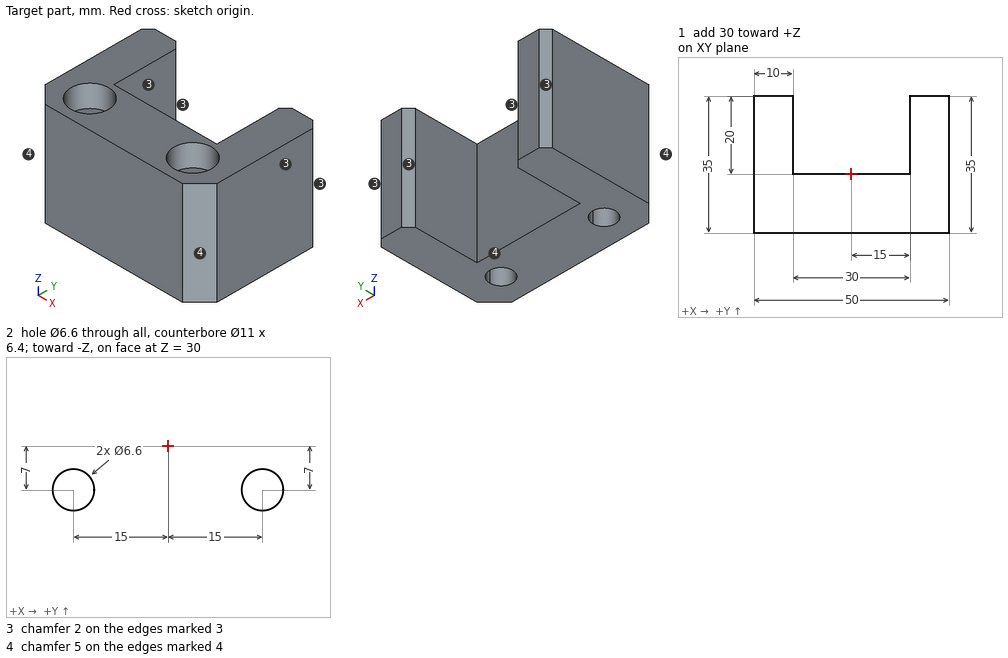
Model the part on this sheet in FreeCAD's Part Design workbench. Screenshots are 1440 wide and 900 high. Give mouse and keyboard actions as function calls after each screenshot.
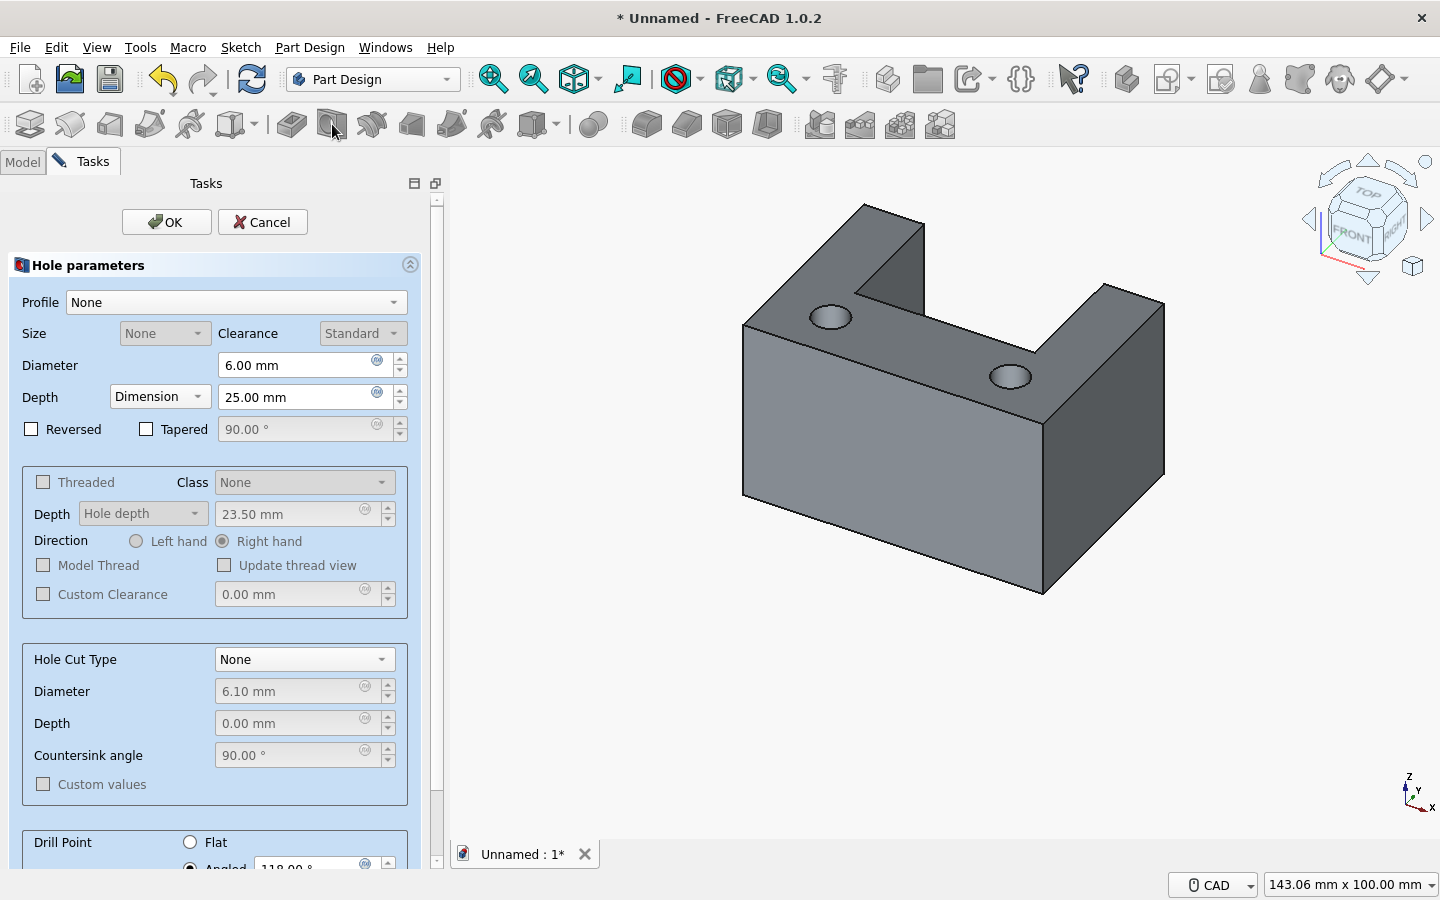
triple_click(305, 365)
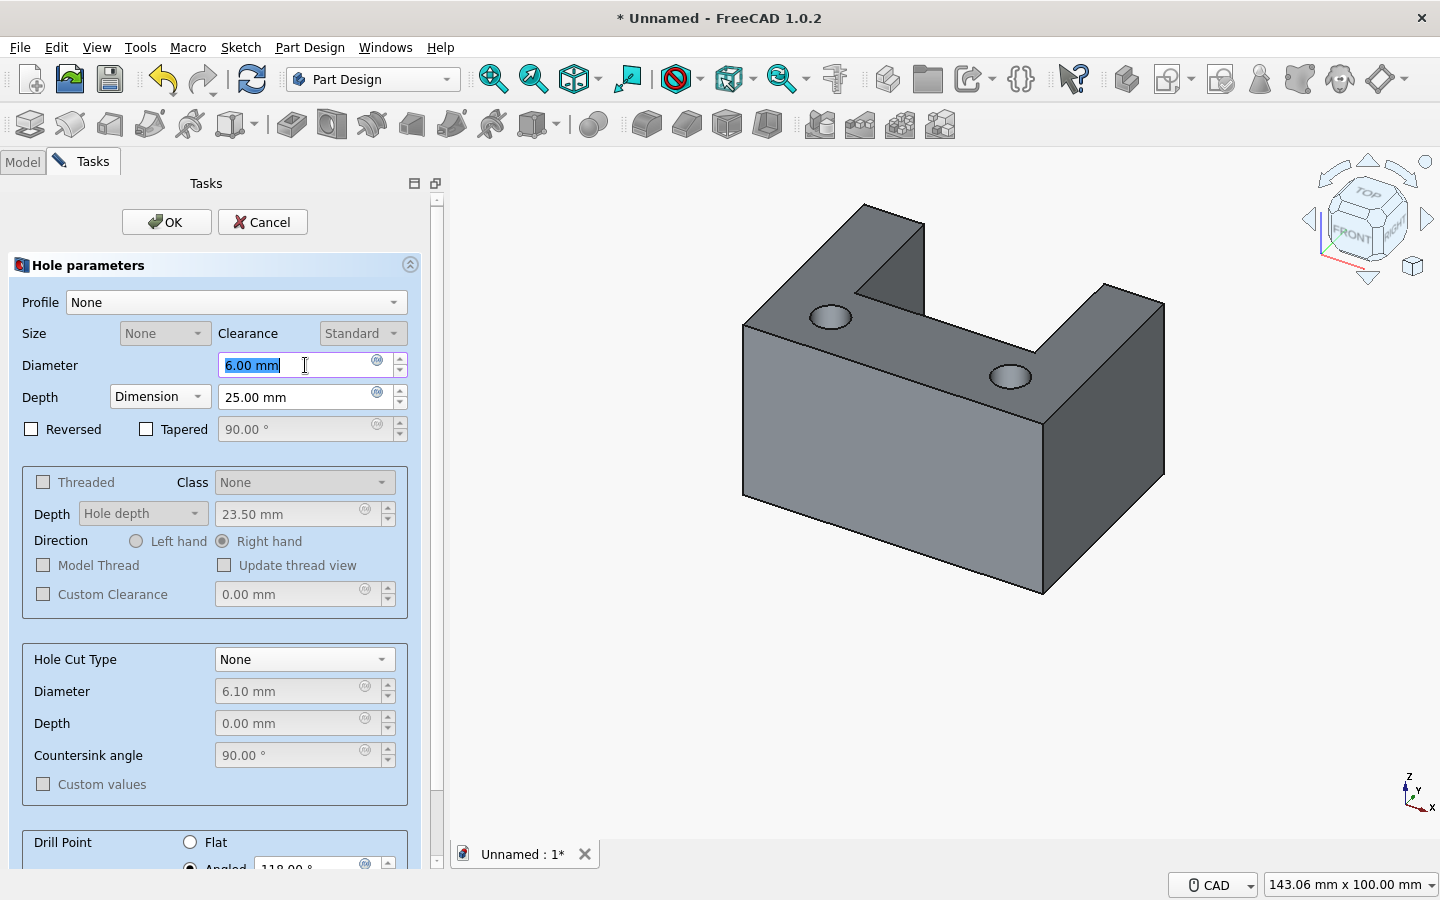
text(6.6)
key(Tab)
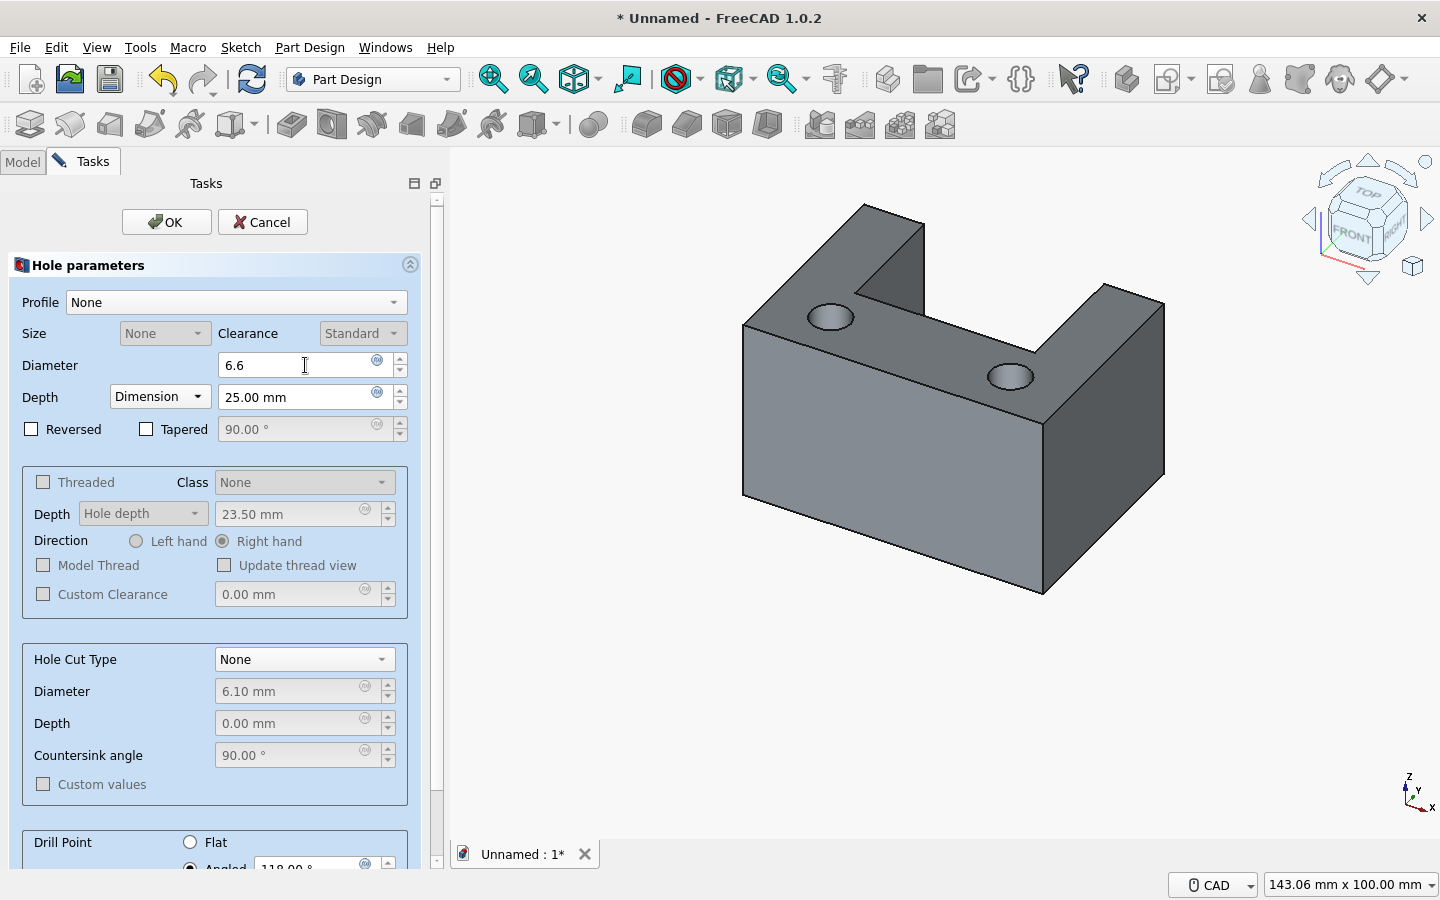
click(161, 396)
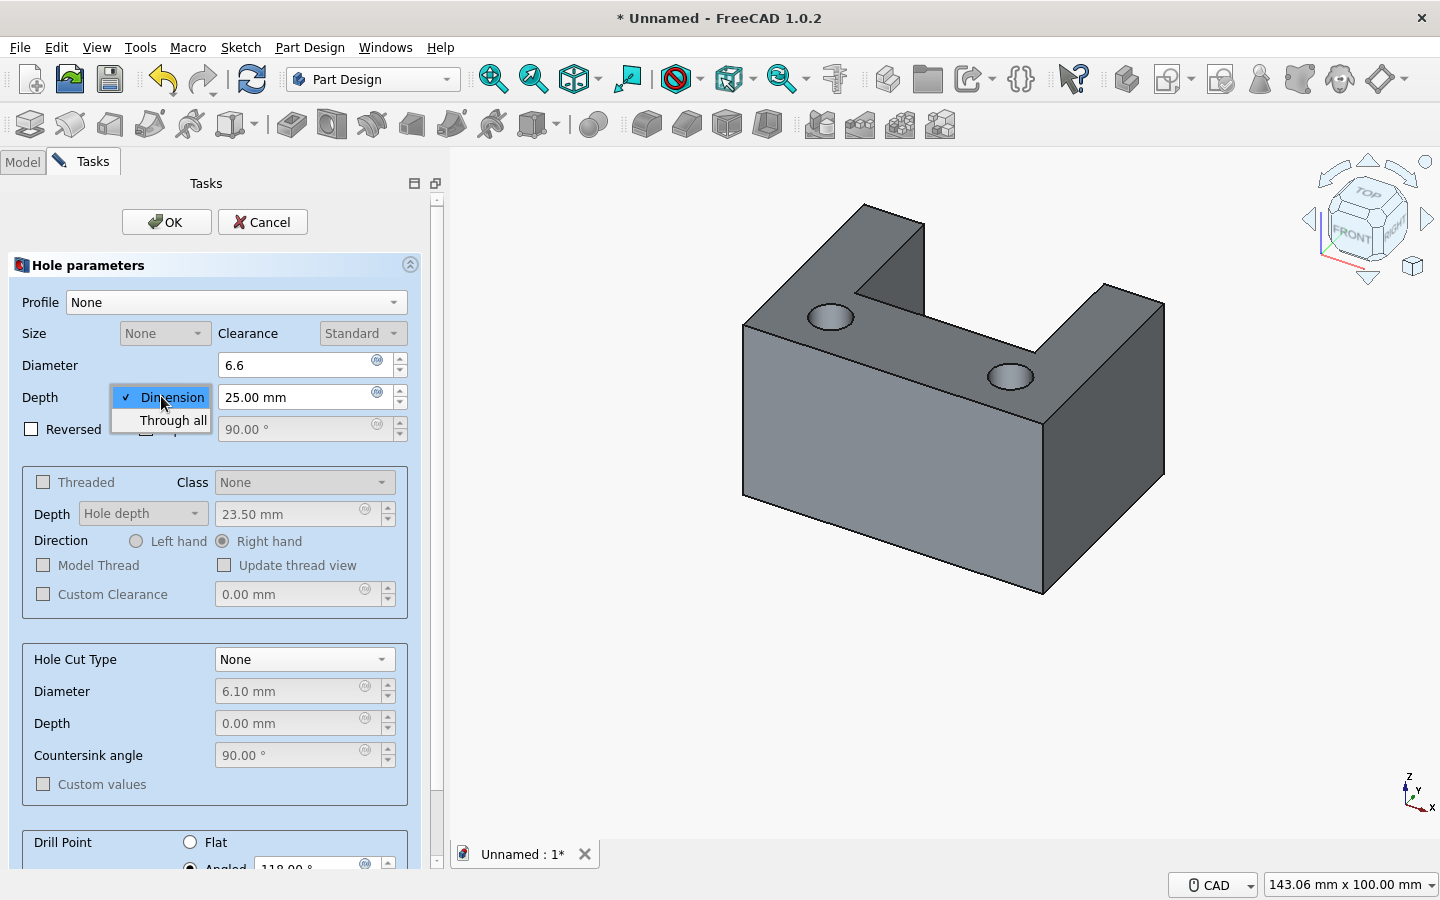
click(160, 420)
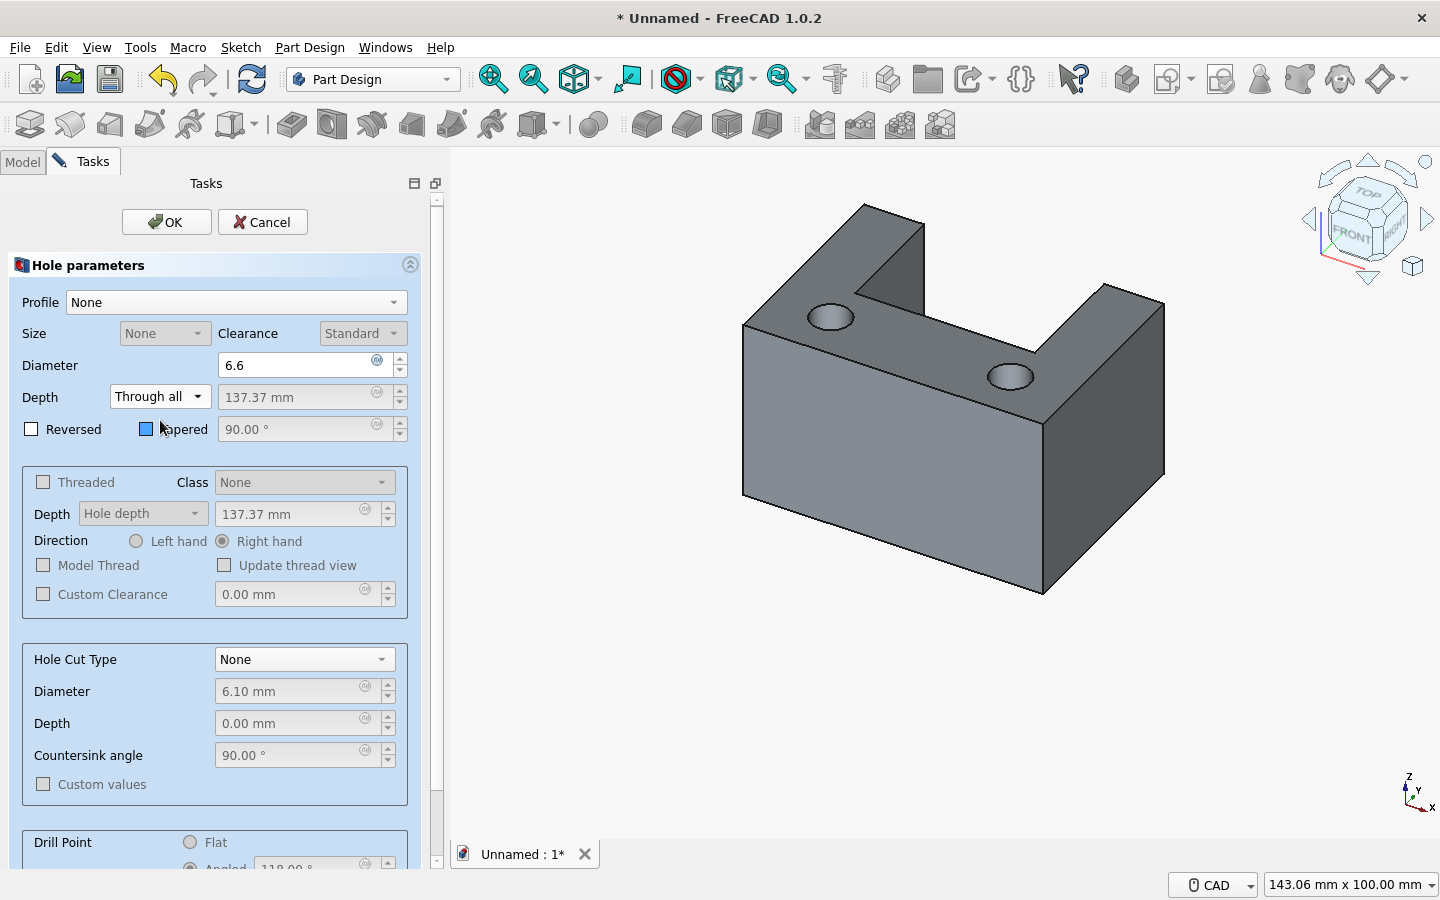
click(306, 660)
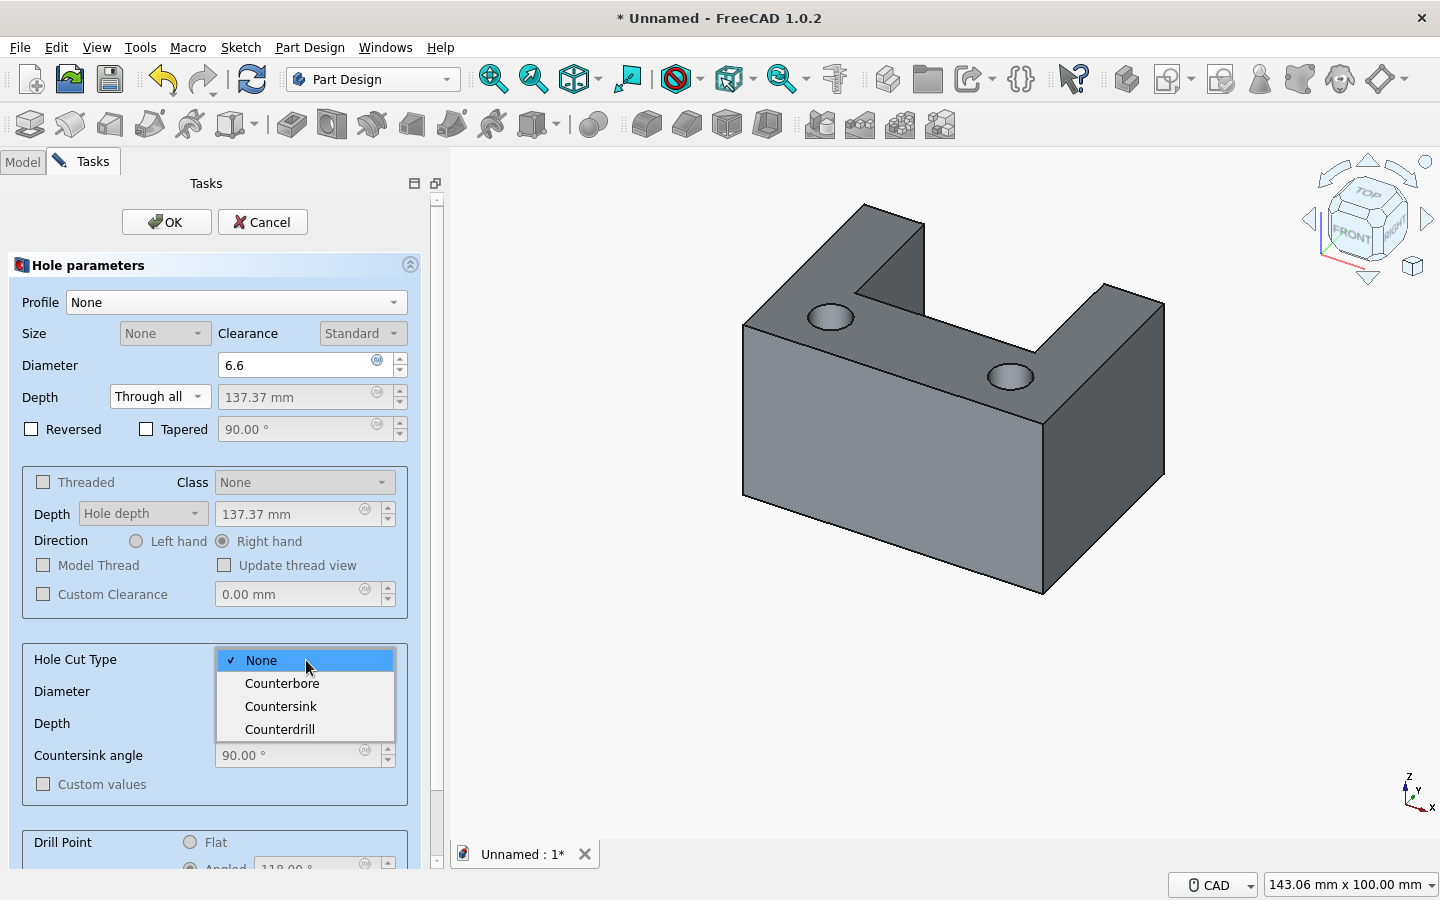
click(304, 684)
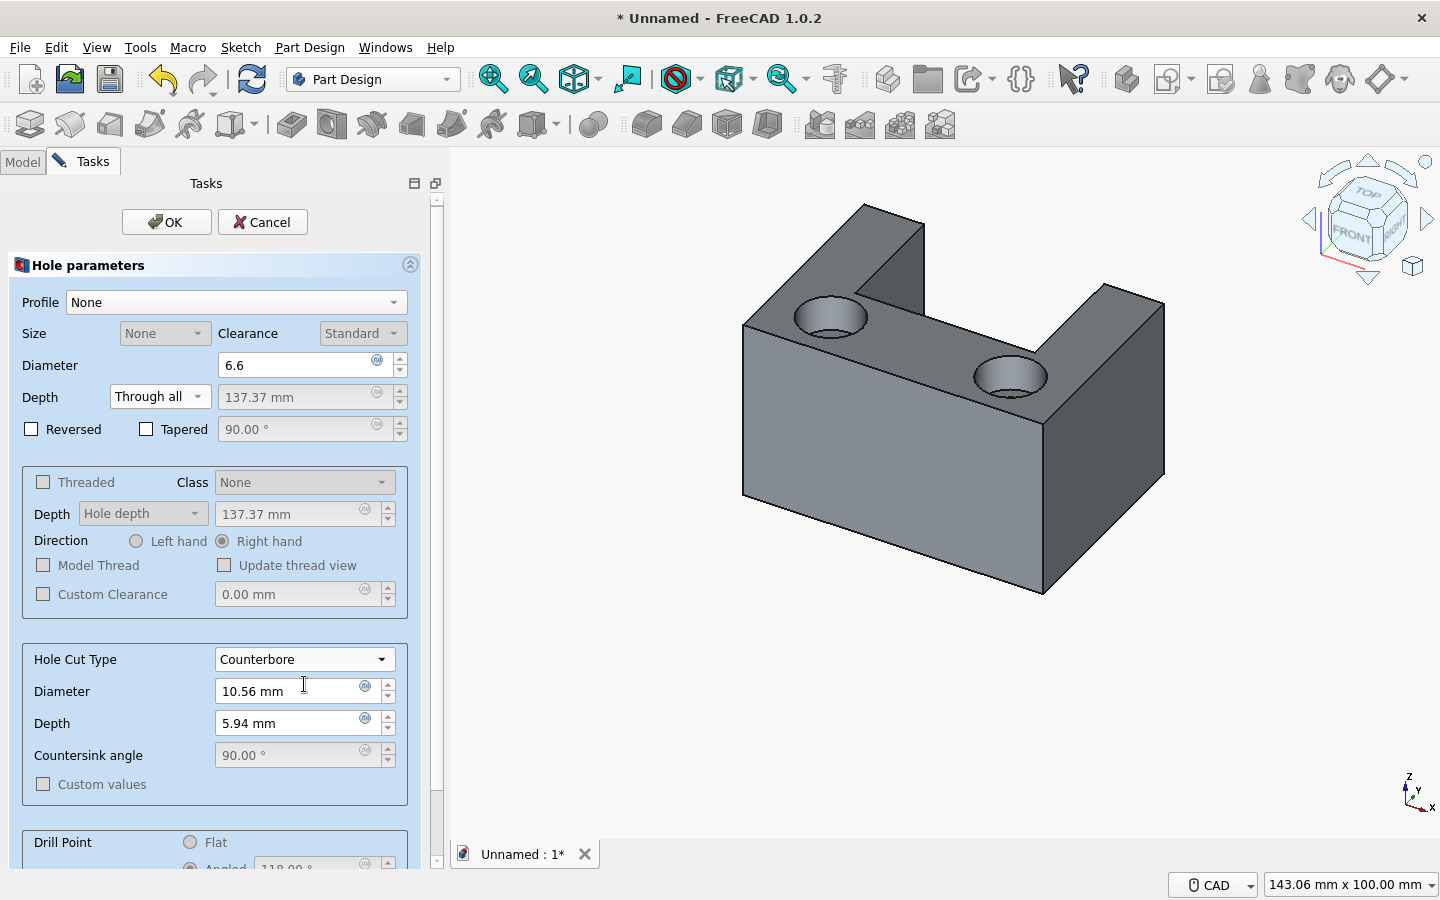
triple_click(298, 691)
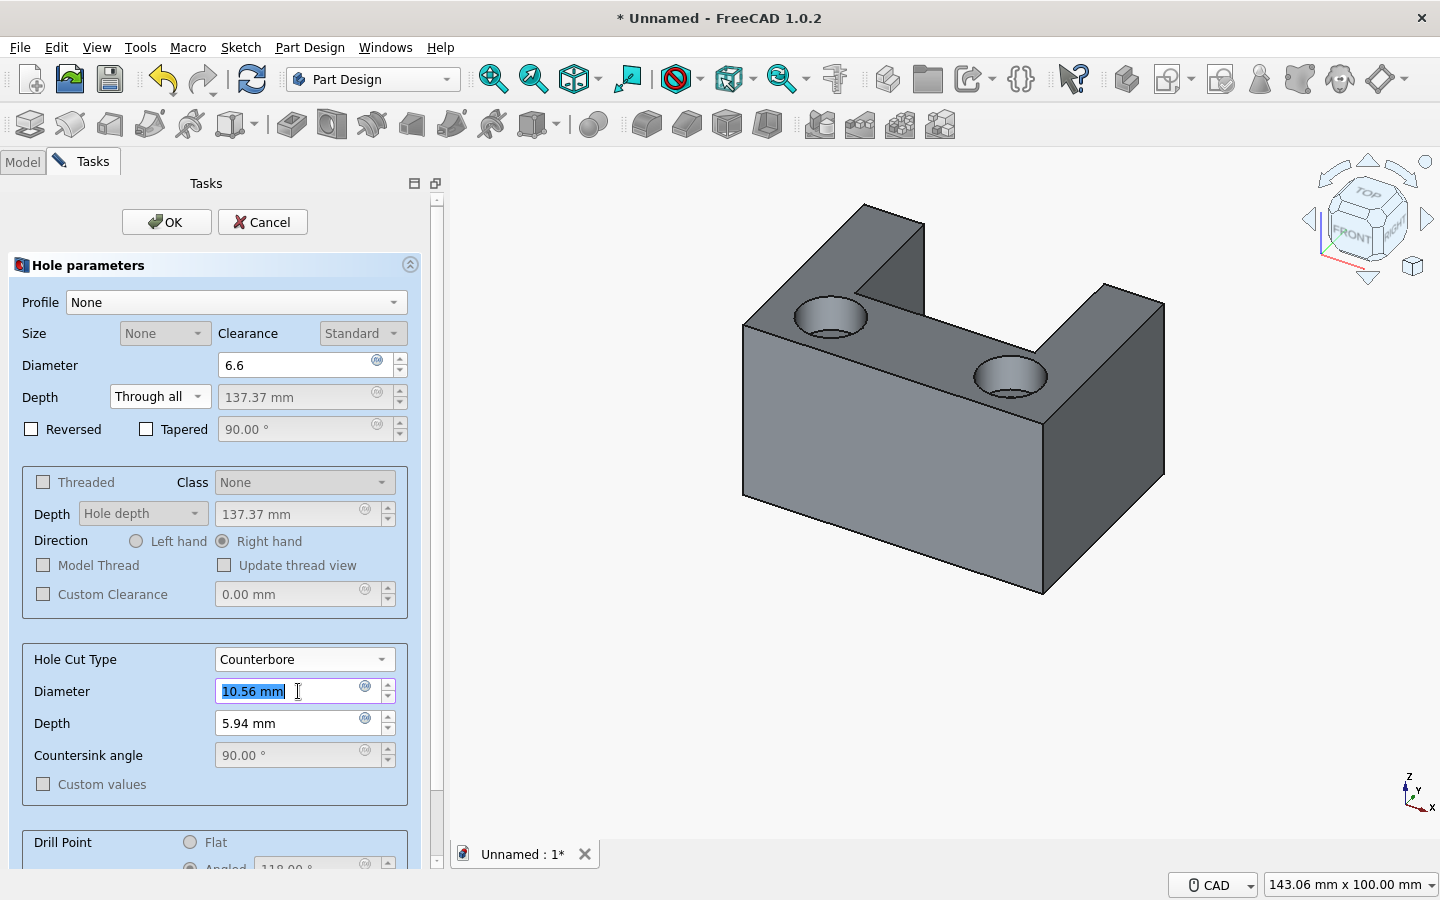
text(11)
key(Tab)